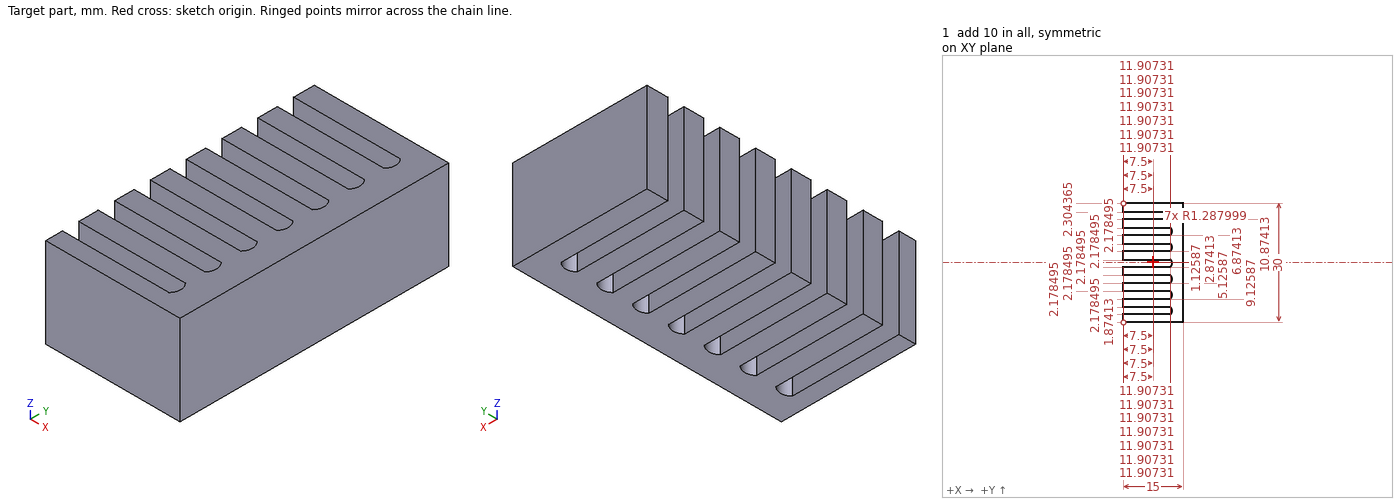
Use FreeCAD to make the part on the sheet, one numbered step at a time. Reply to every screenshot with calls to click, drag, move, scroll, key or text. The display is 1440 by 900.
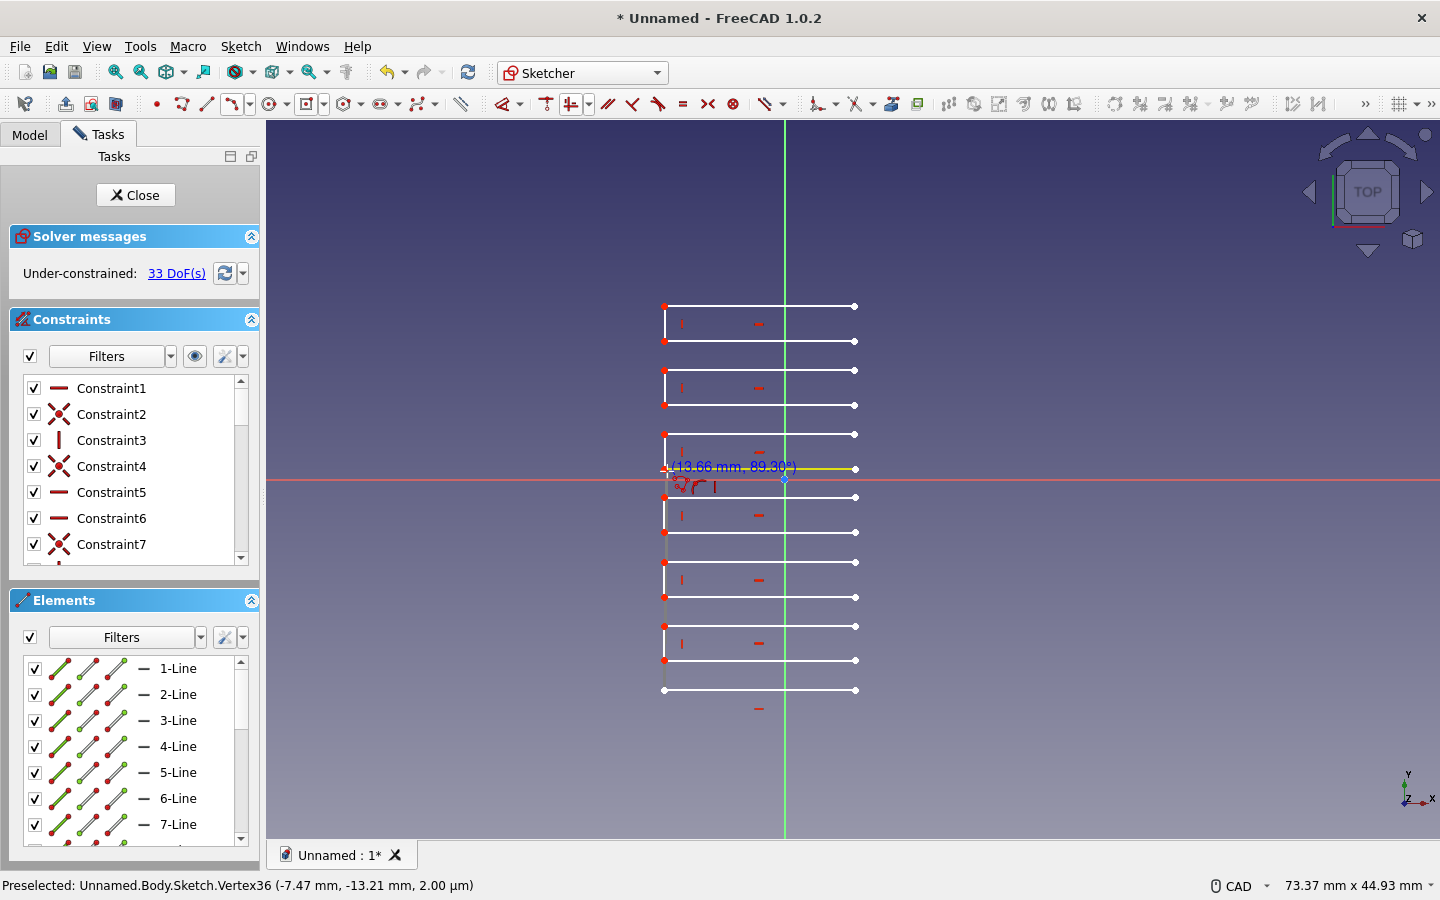
click(664, 720)
click(905, 720)
click(905, 240)
click(665, 240)
click(665, 276)
click(855, 276)
right_click(855, 276)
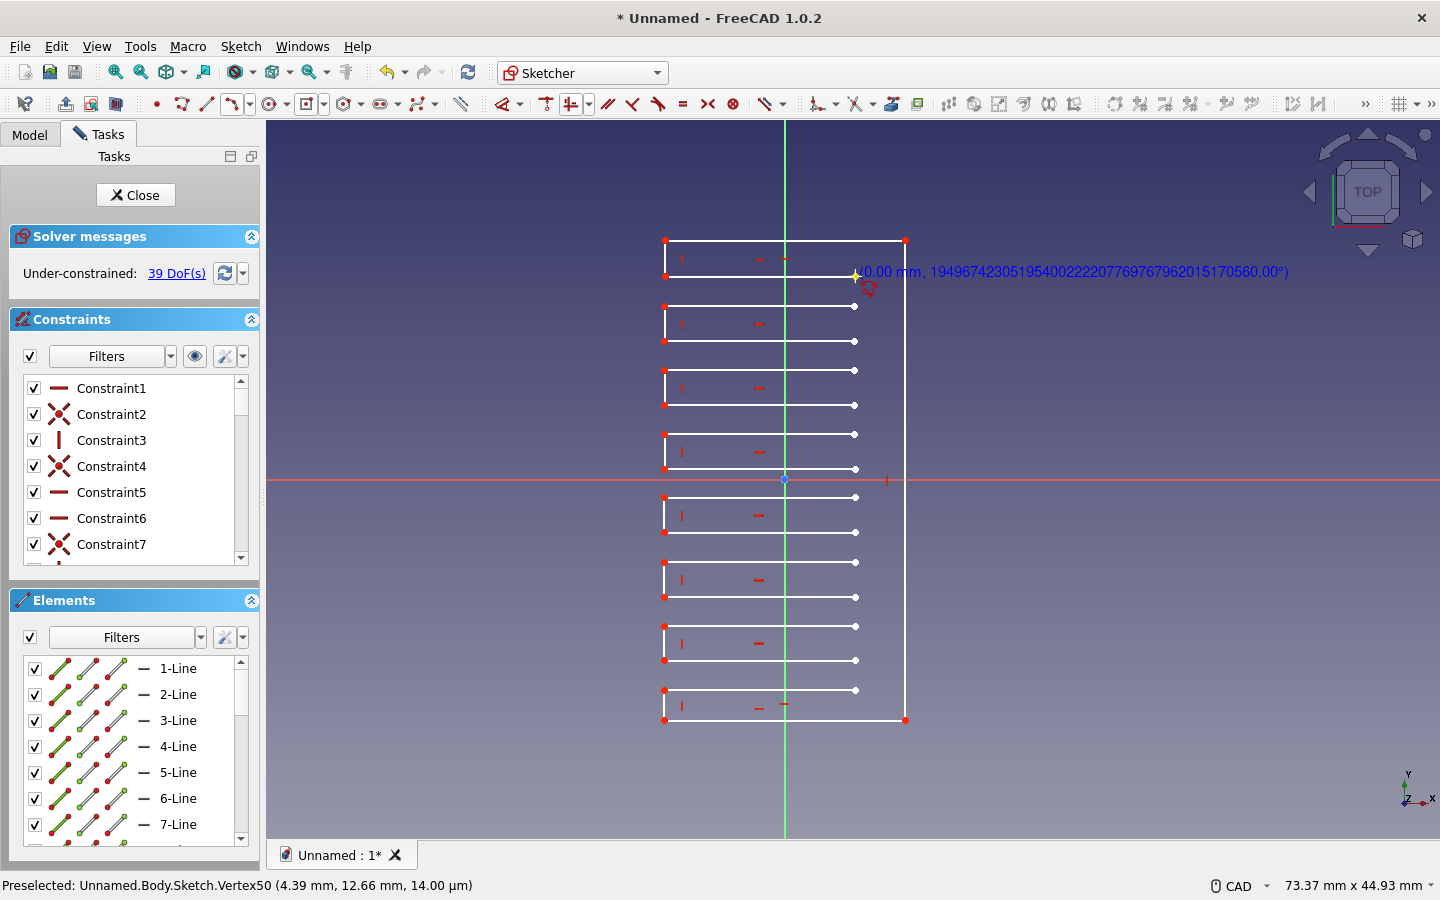
click(232, 104)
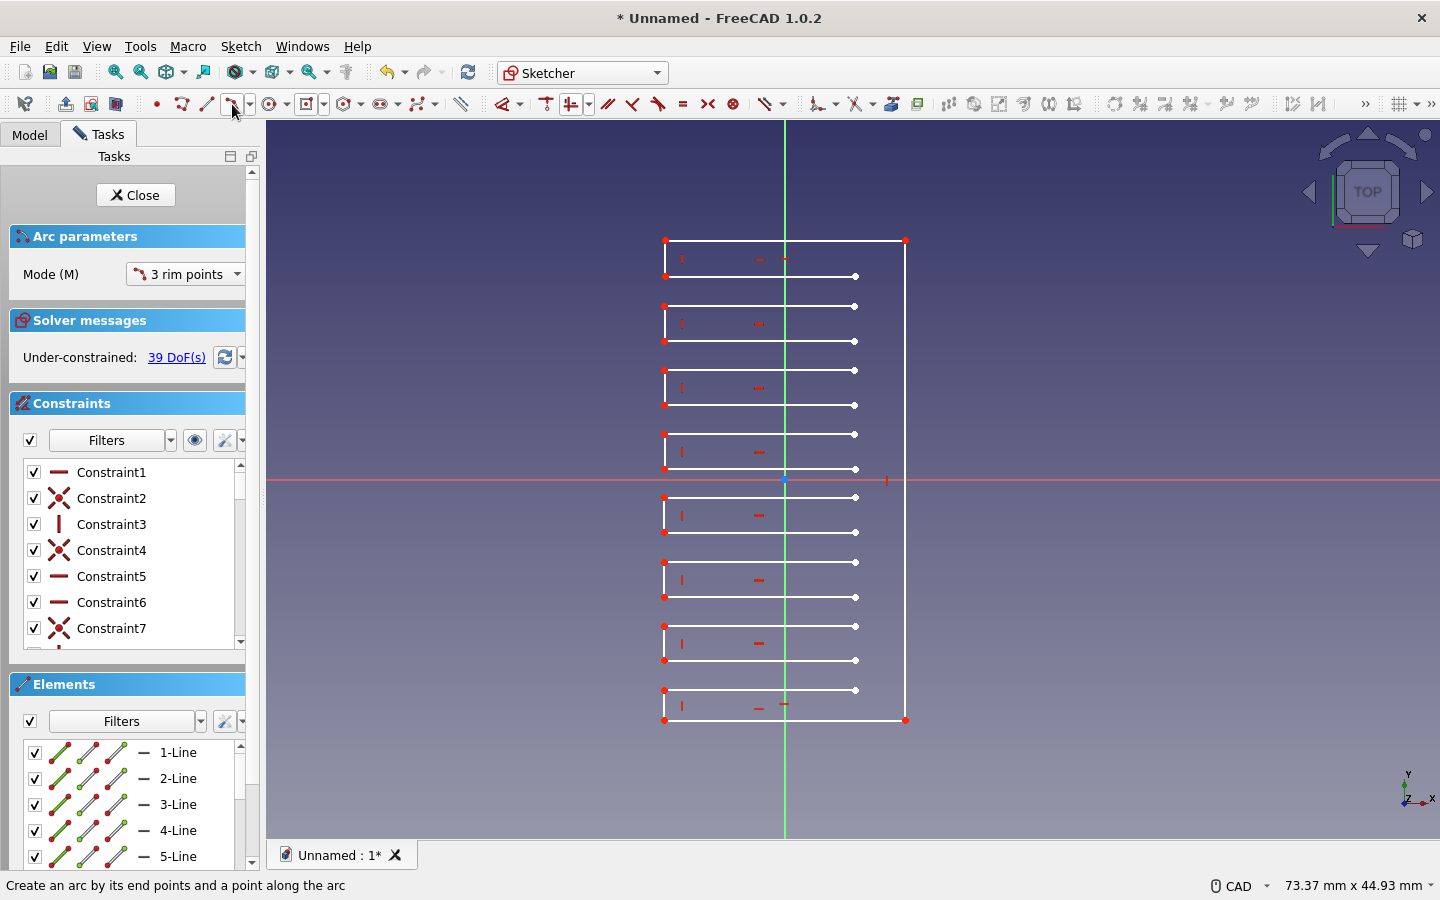
click(855, 341)
click(855, 370)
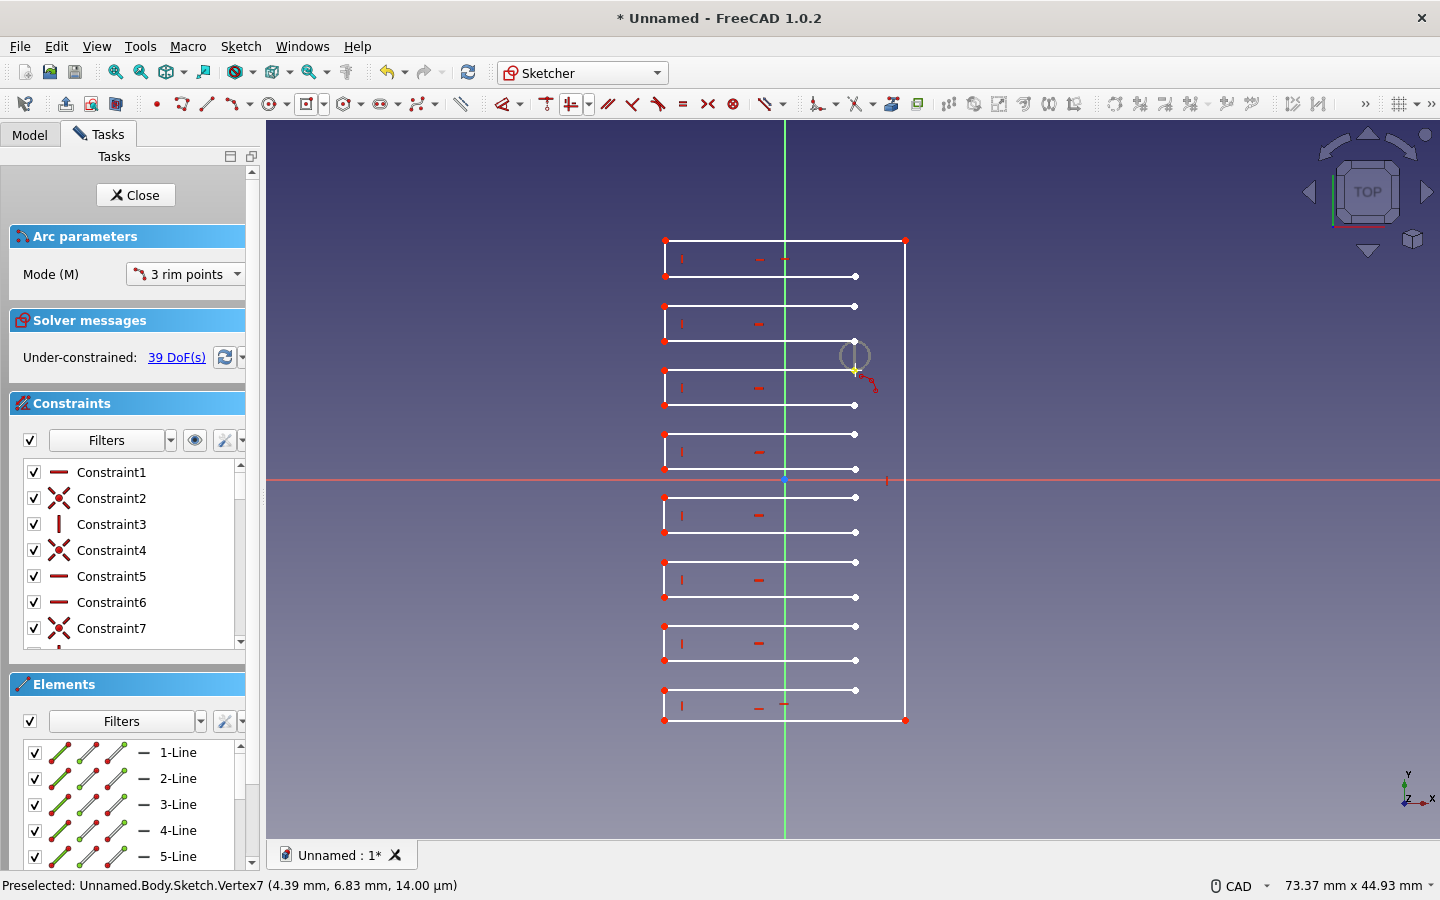
scroll(861, 355, up, 5)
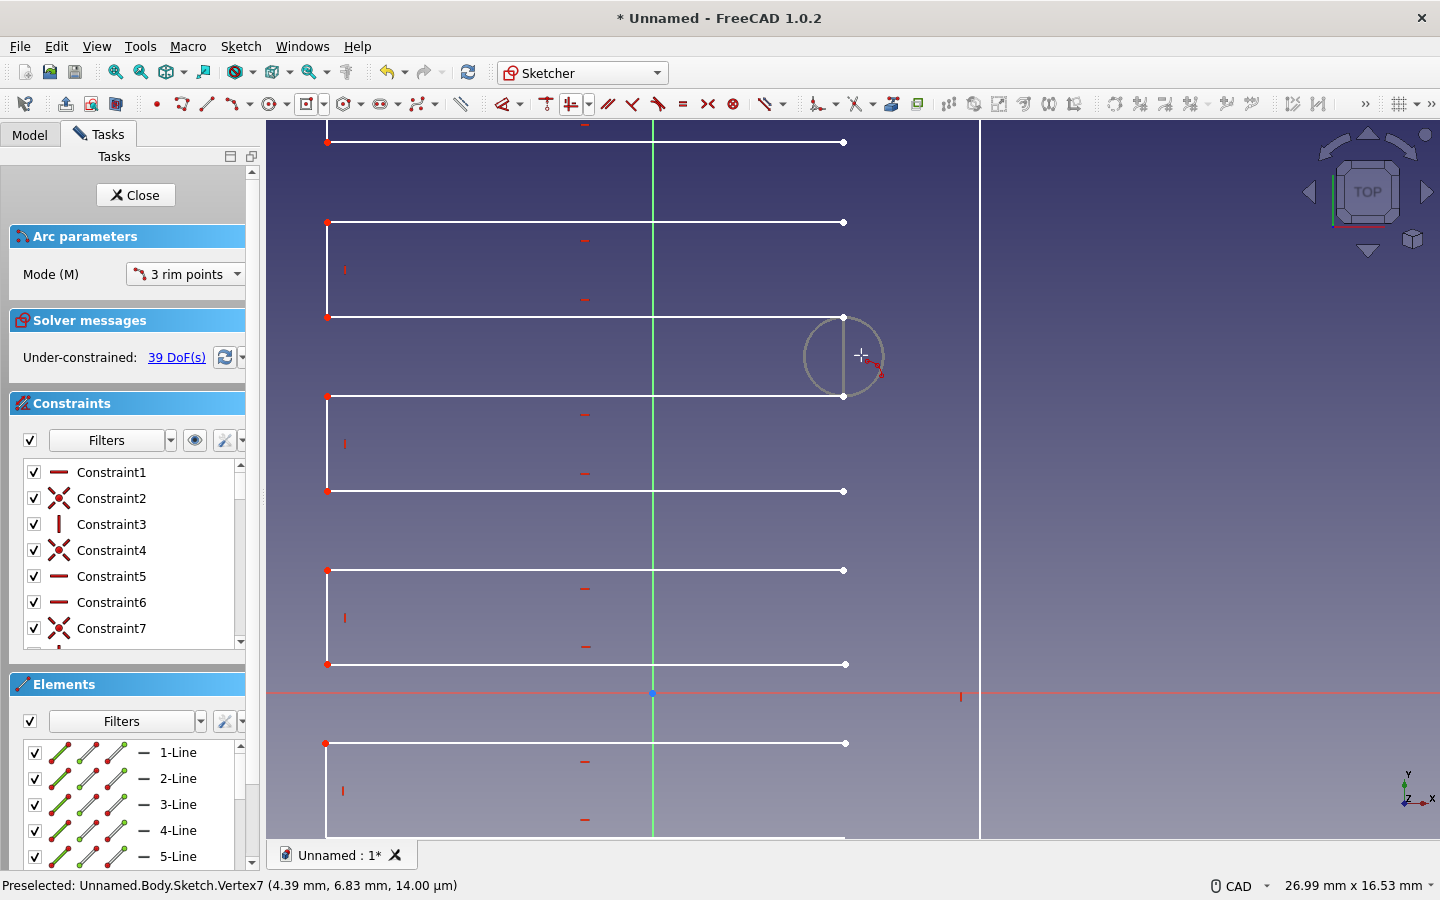
click(861, 354)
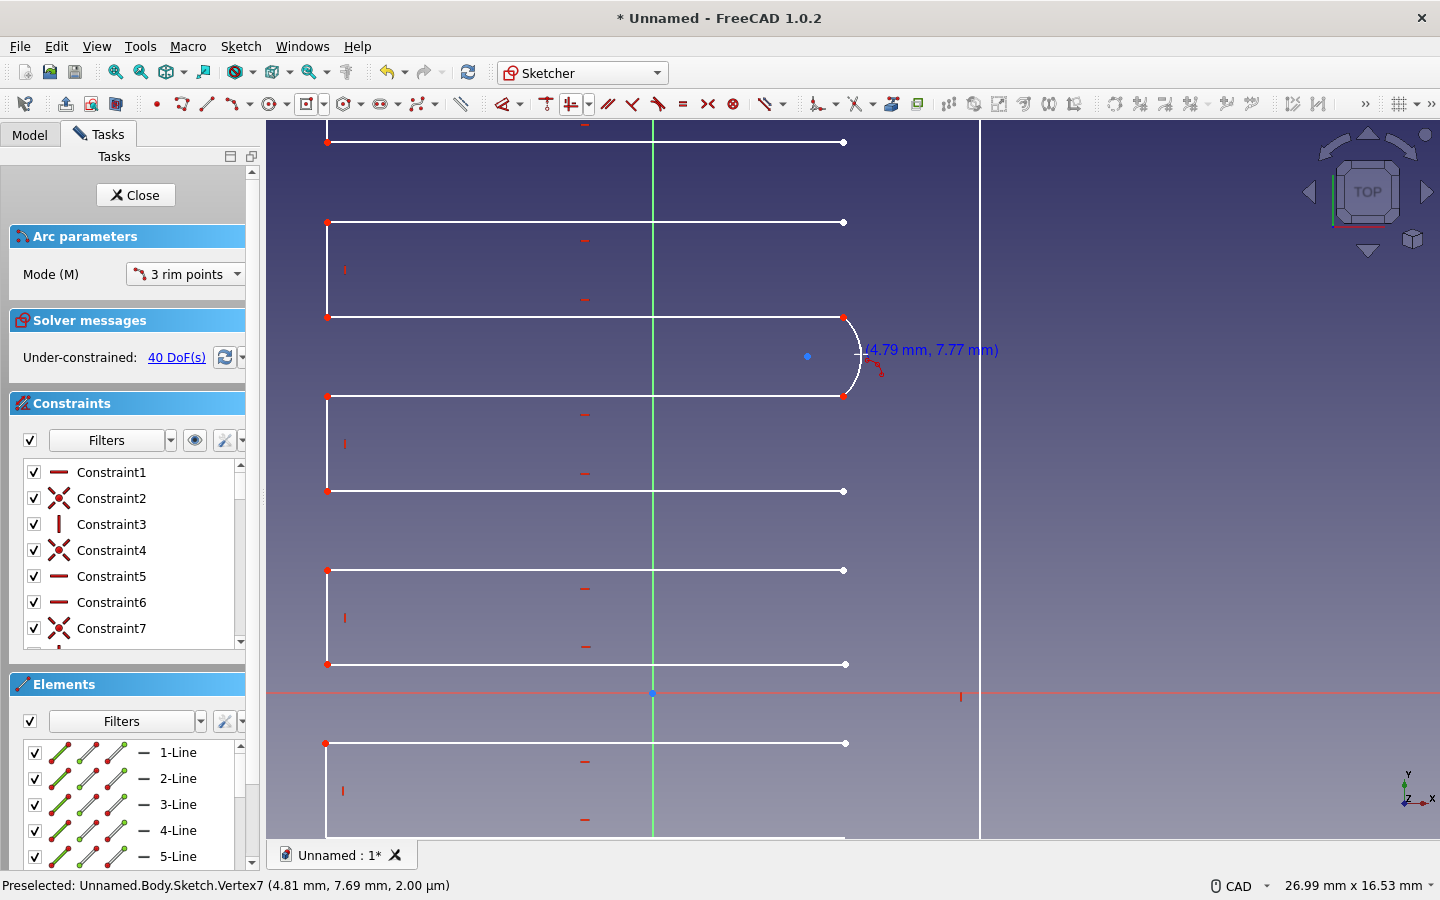
click(844, 491)
click(844, 570)
click(861, 528)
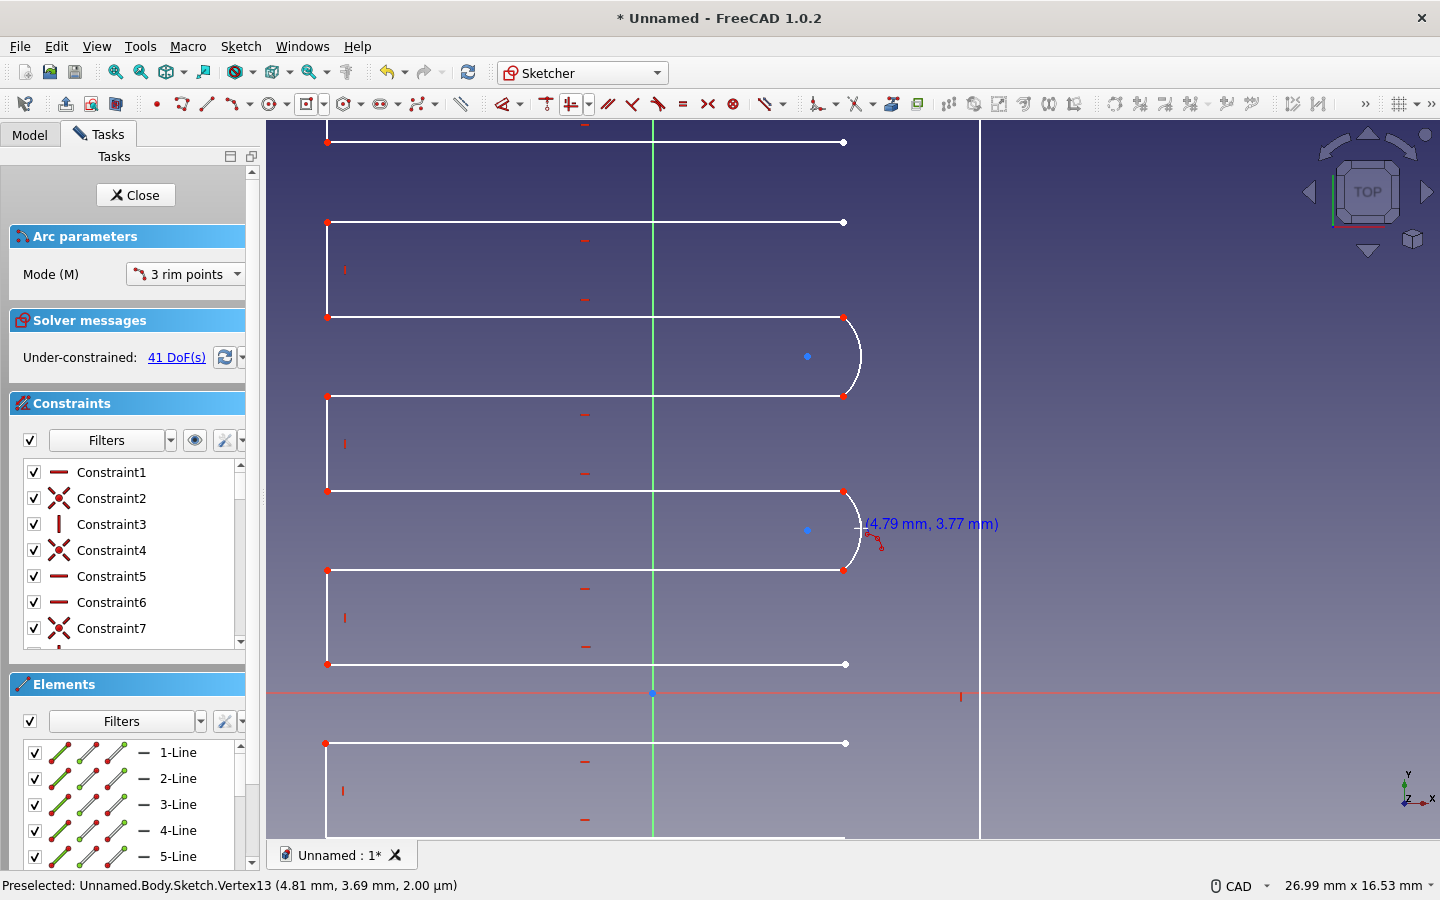
click(845, 665)
click(845, 743)
click(860, 711)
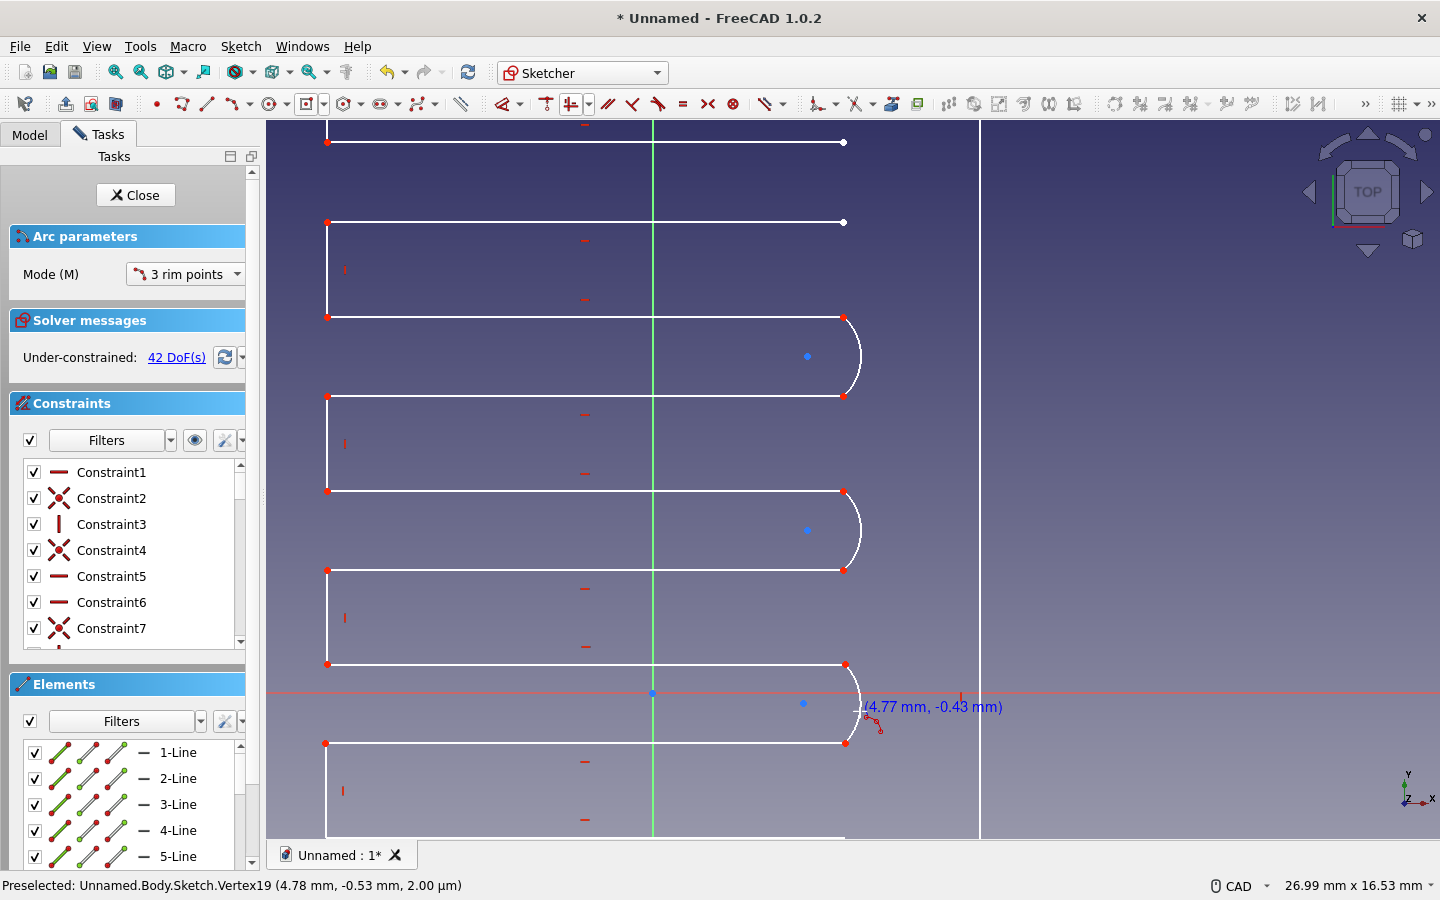
scroll(861, 355, down, 5)